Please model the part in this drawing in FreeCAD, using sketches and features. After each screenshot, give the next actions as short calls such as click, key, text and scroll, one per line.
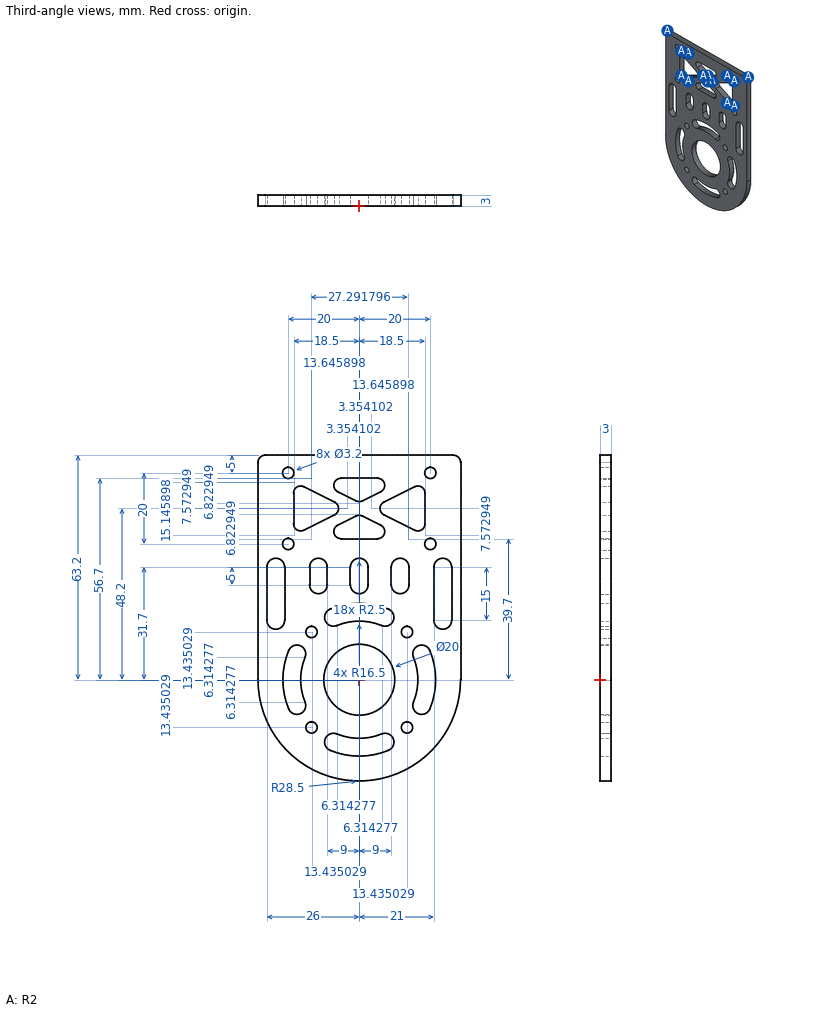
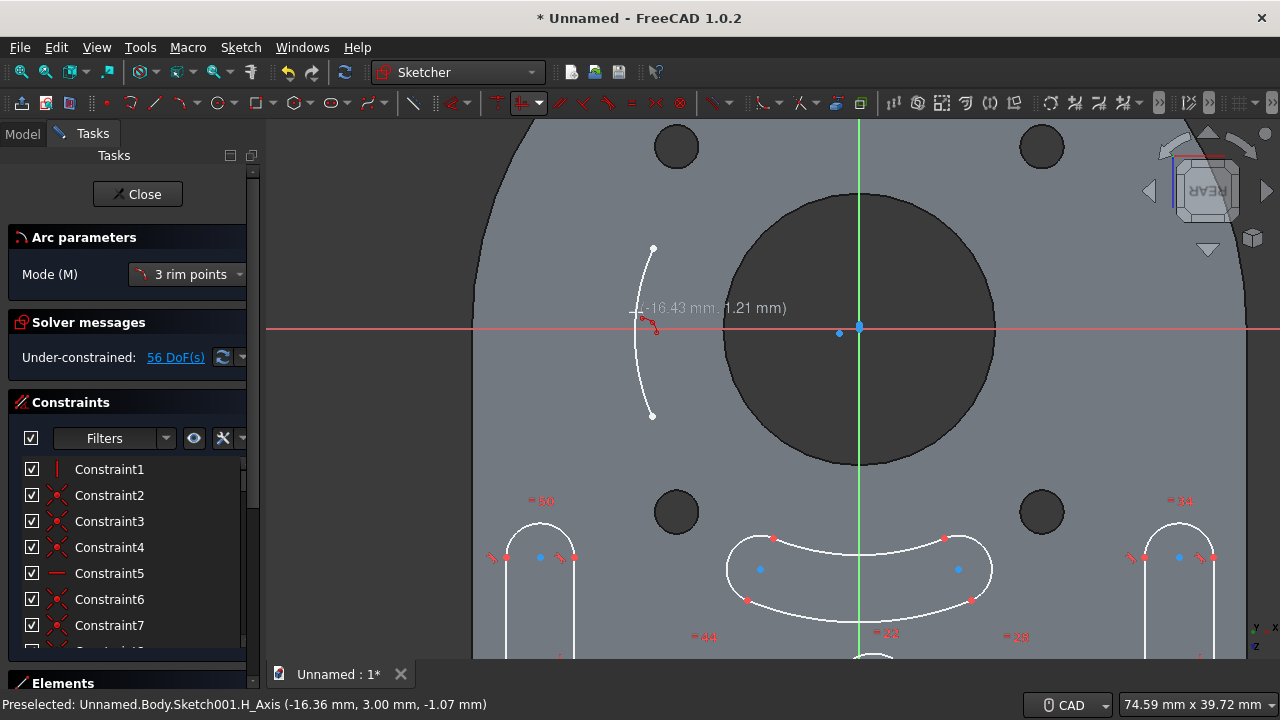
click(654, 248)
click(589, 218)
click(634, 199)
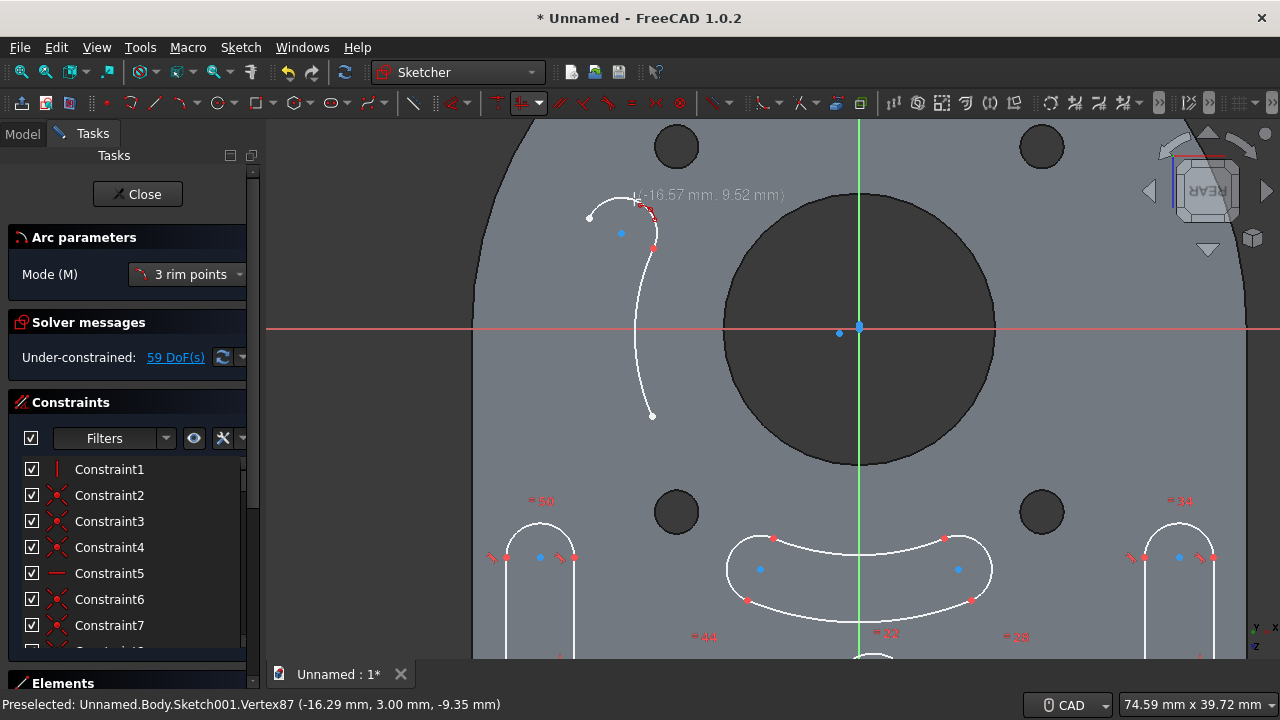
click(589, 219)
click(589, 441)
click(568, 306)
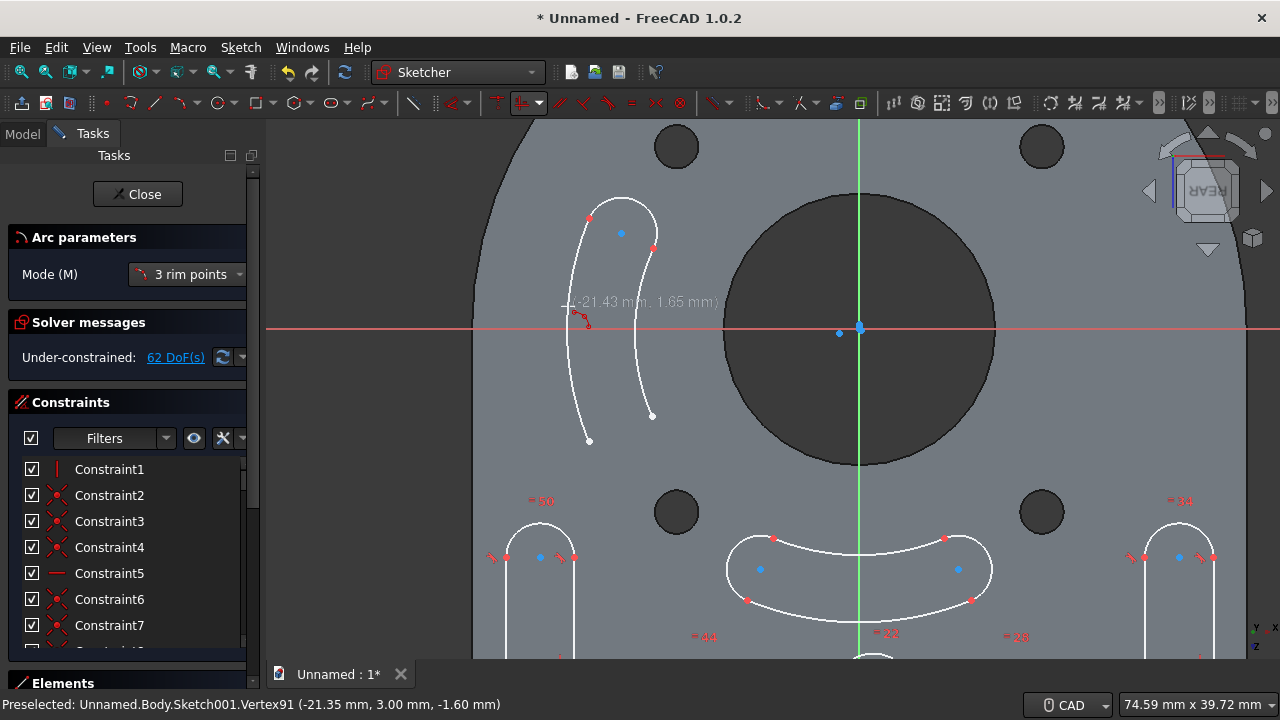
click(589, 442)
click(652, 416)
click(634, 460)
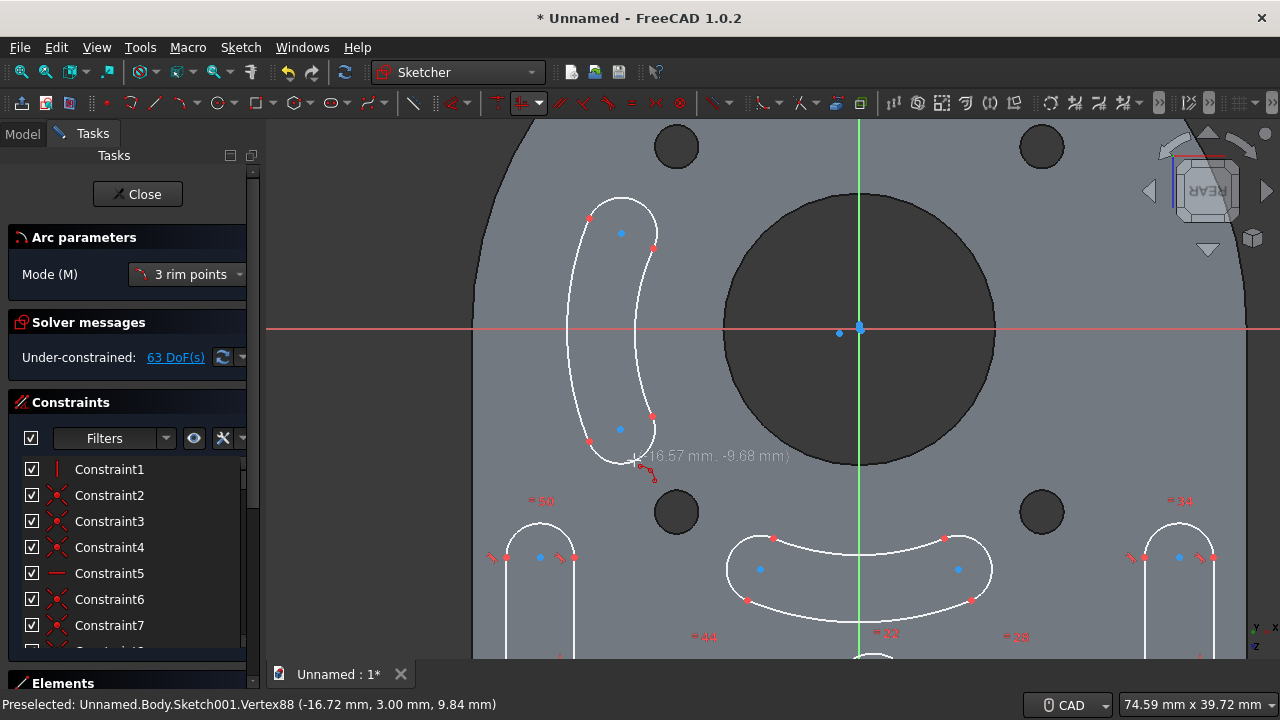
click(1067, 244)
click(1067, 415)
click(1083, 347)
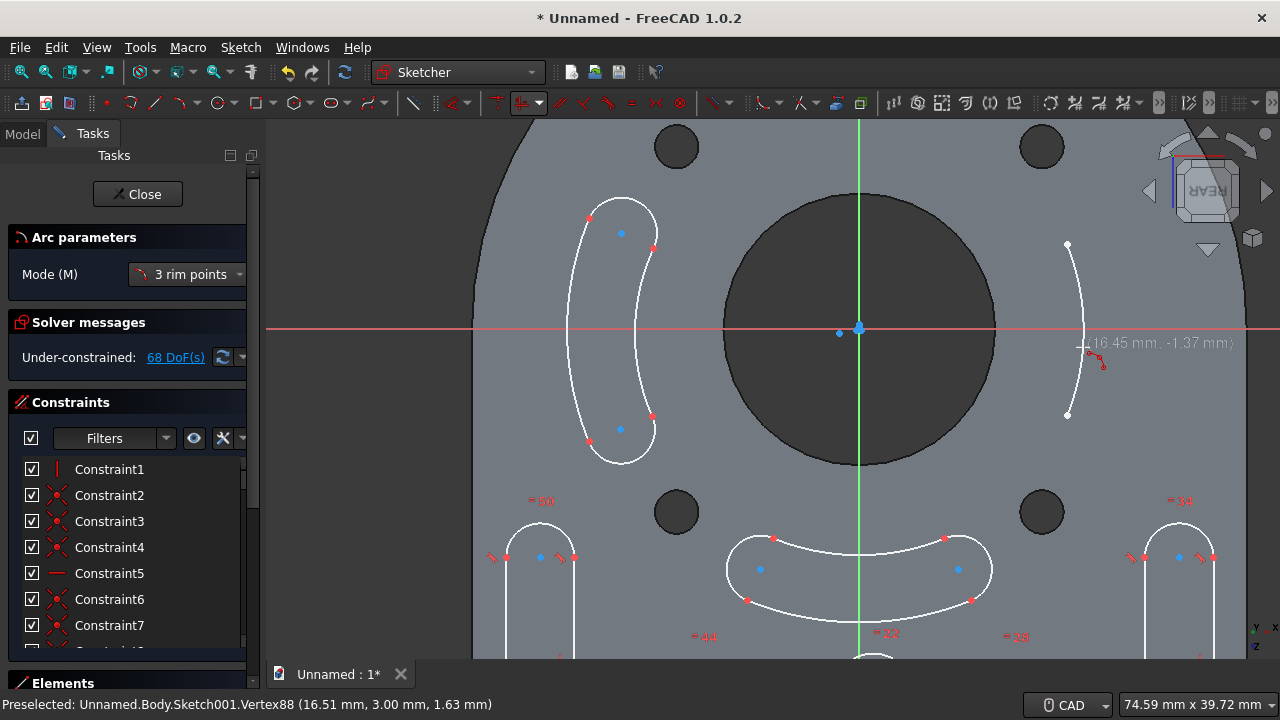
click(1067, 416)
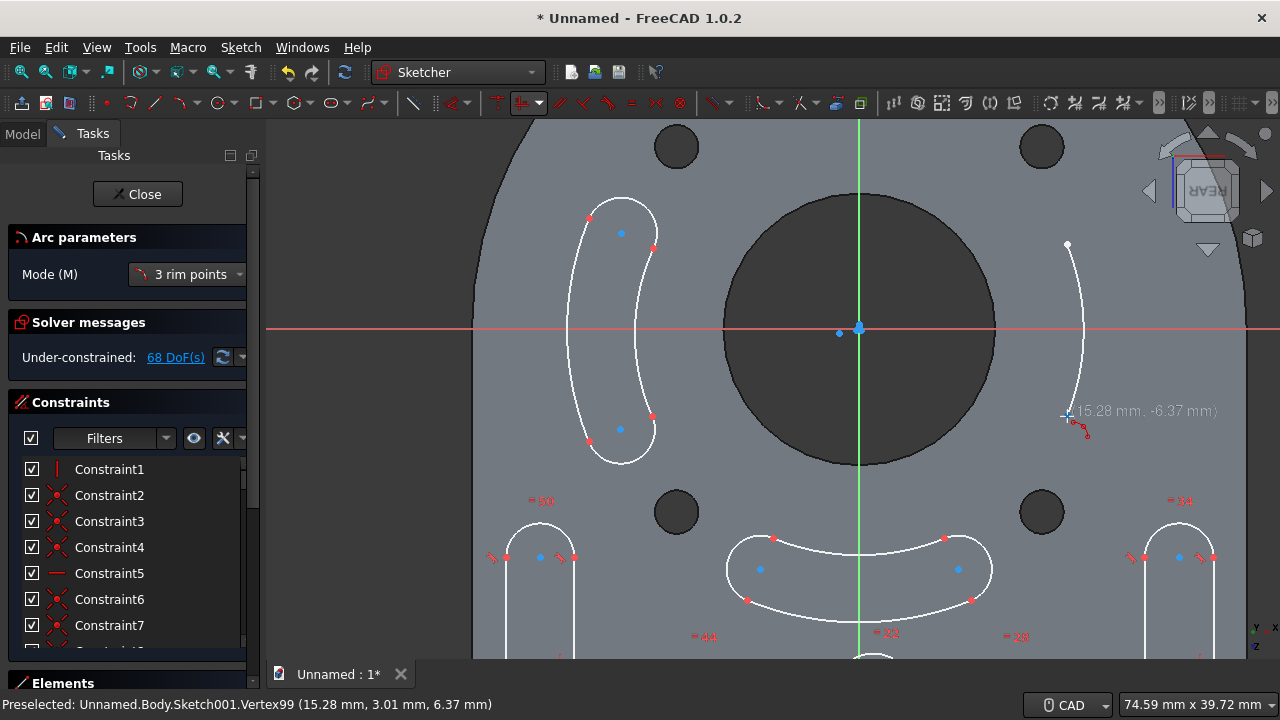
scroll(638, 312, down, 6)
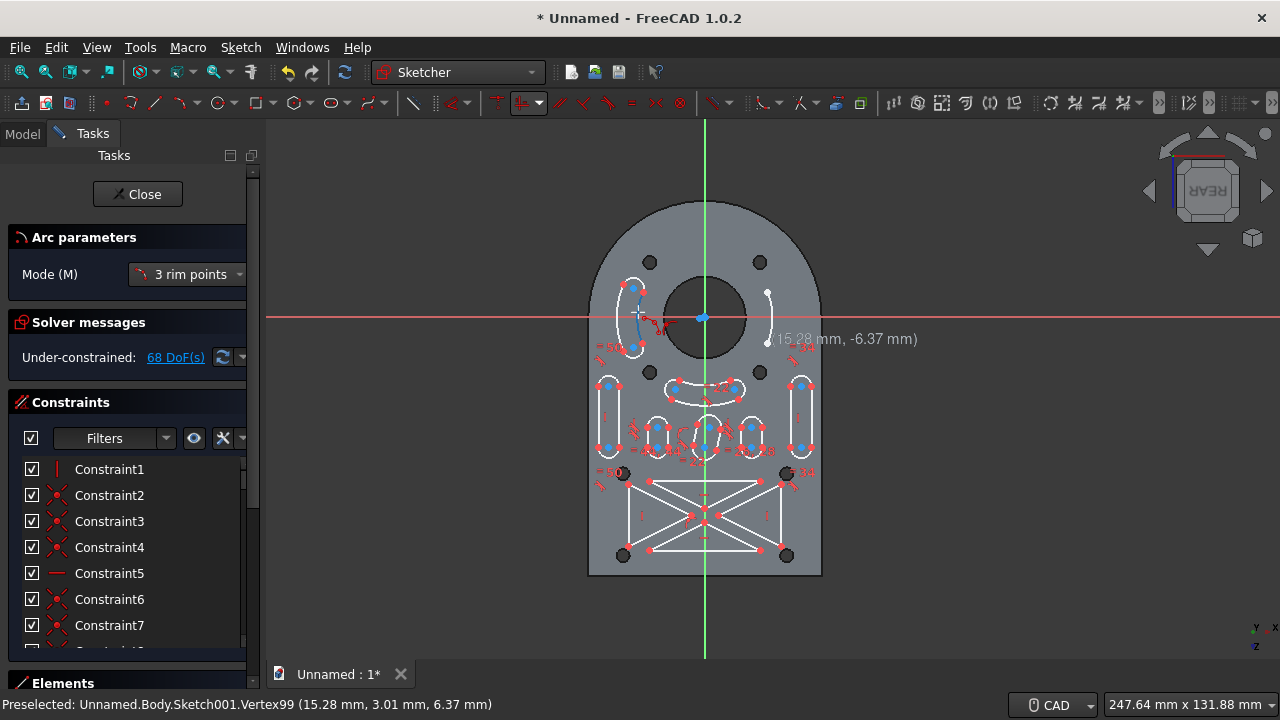
click(786, 351)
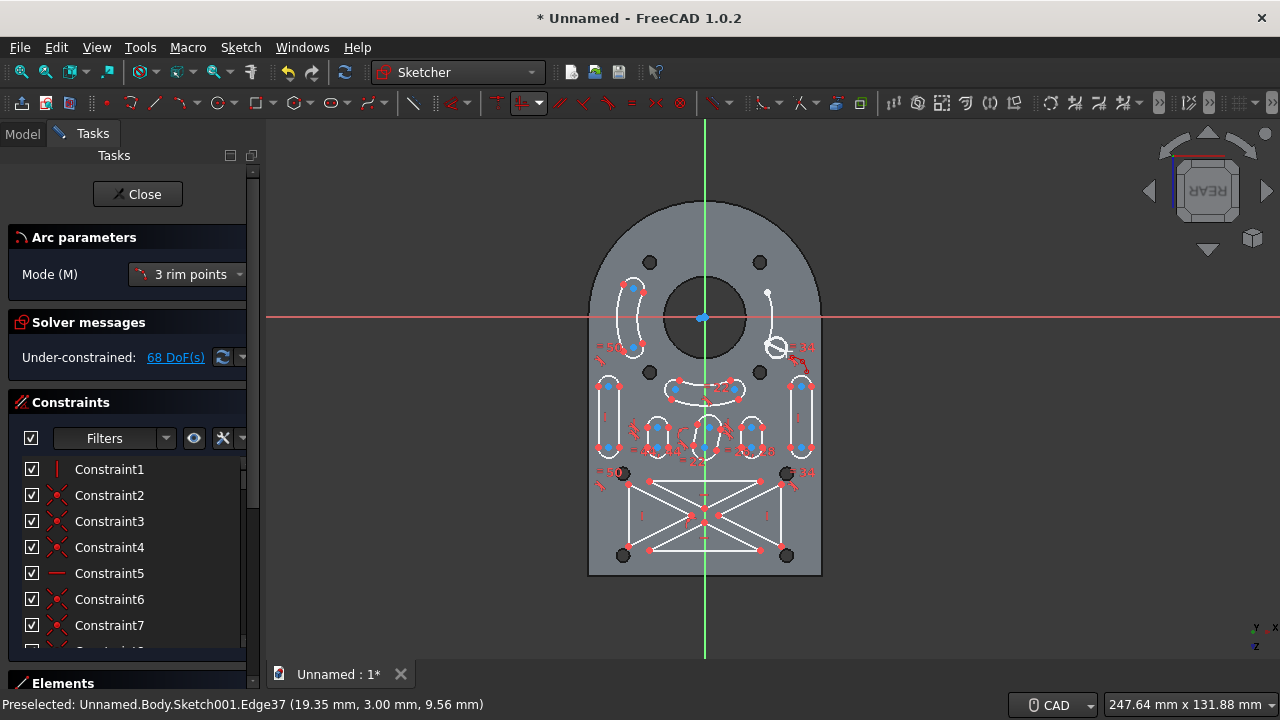
scroll(773, 357, up, 3)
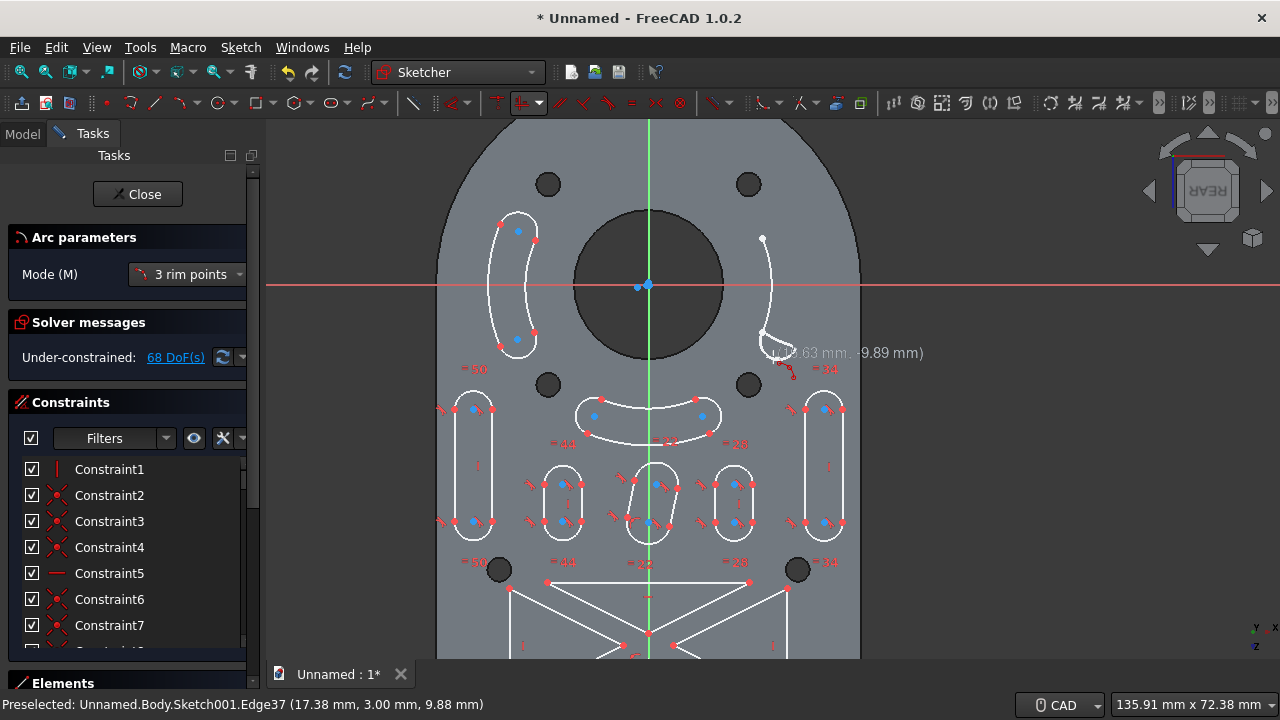
click(772, 356)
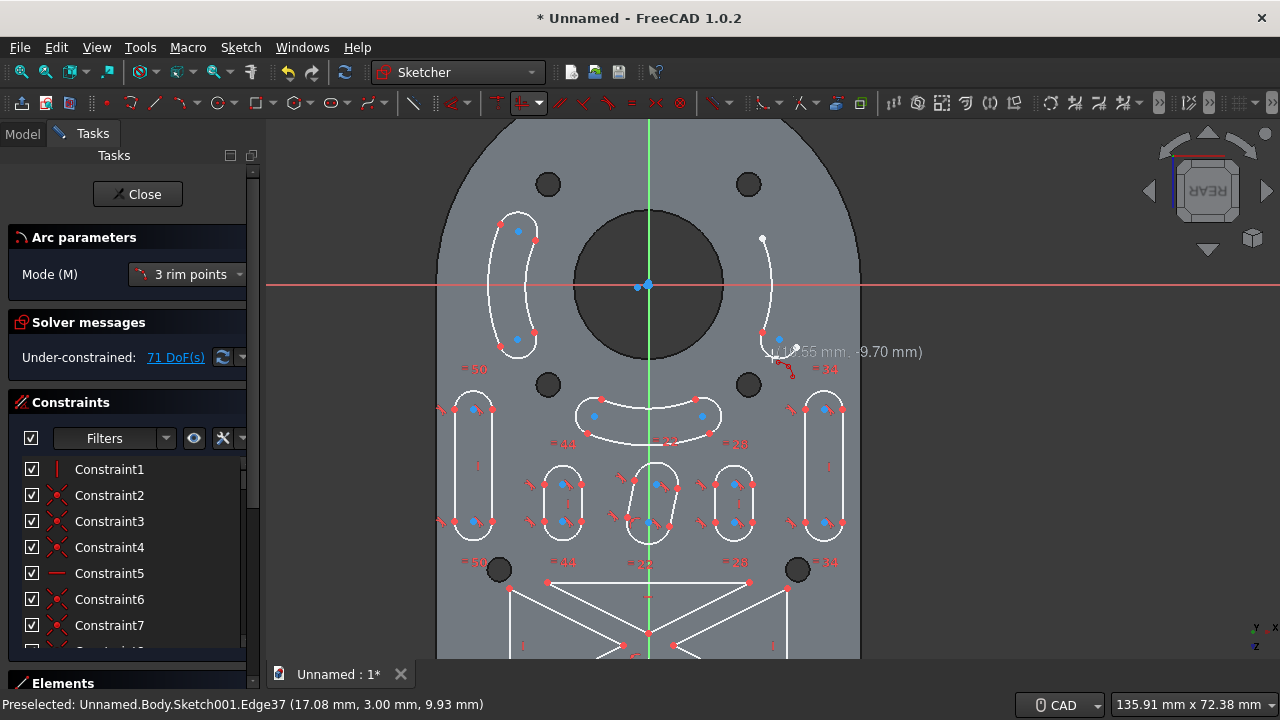
click(796, 348)
click(797, 223)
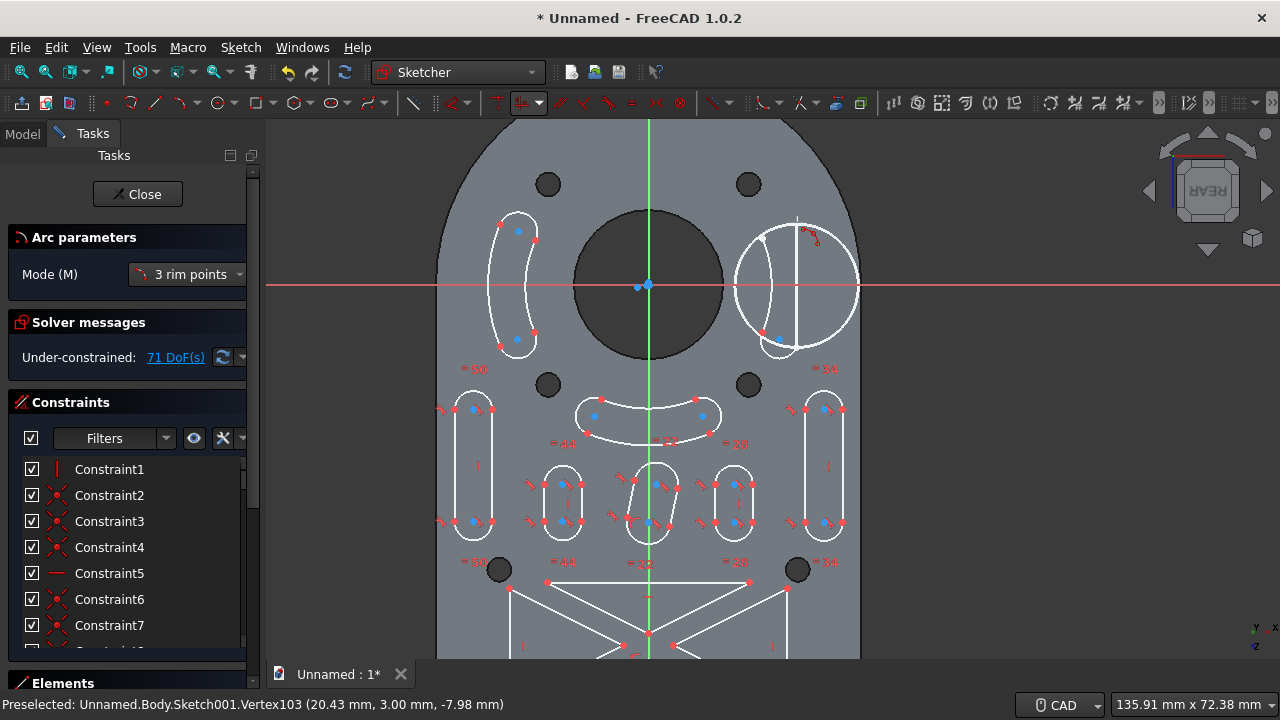
scroll(808, 297, up, 2)